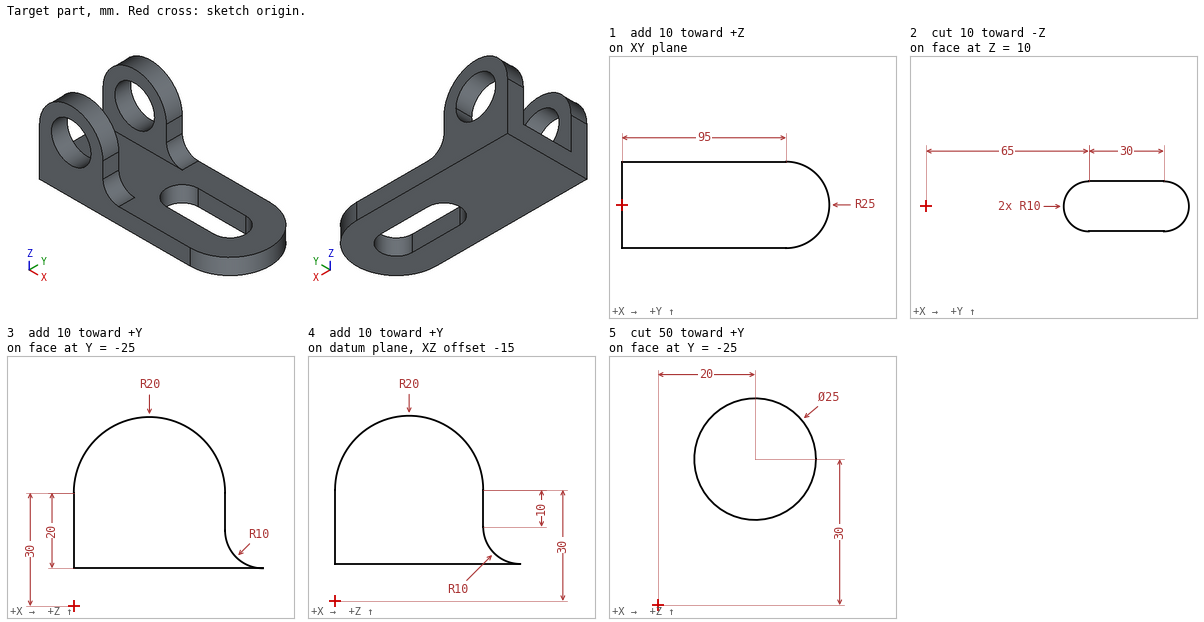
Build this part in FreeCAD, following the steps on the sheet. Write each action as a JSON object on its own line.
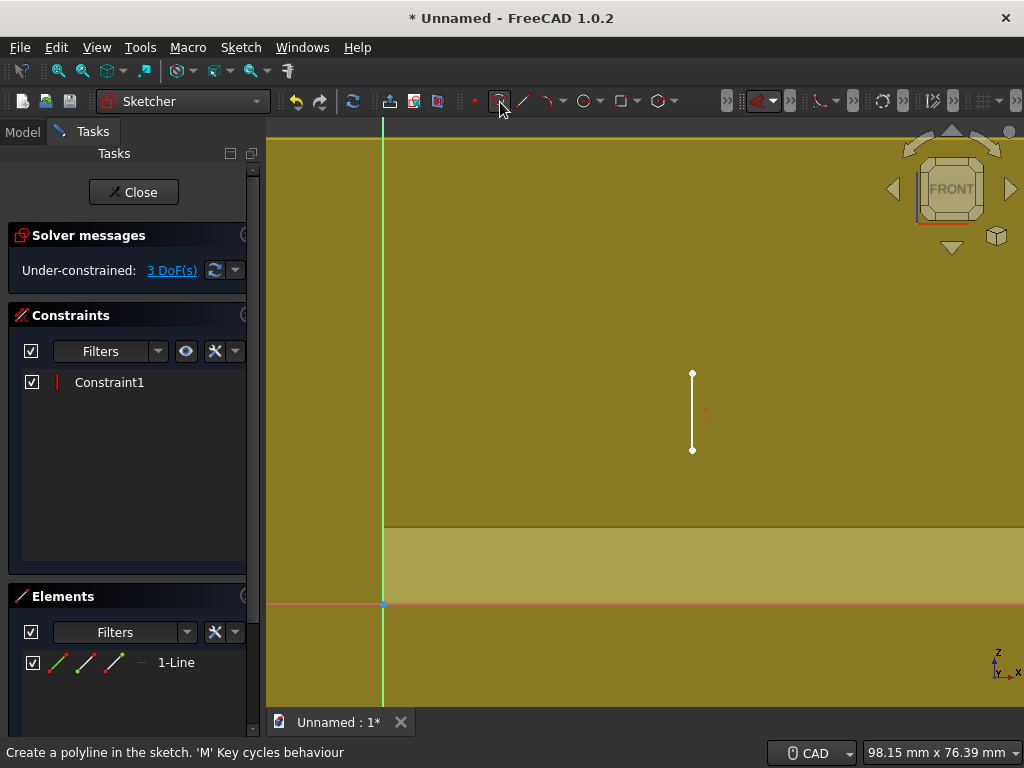
{"action": "left_click", "coordinate": [769, 527]}
{"action": "left_click", "coordinate": [383, 527]}
{"action": "left_click", "coordinate": [392, 373]}
{"action": "right_click", "coordinate": [392, 373]}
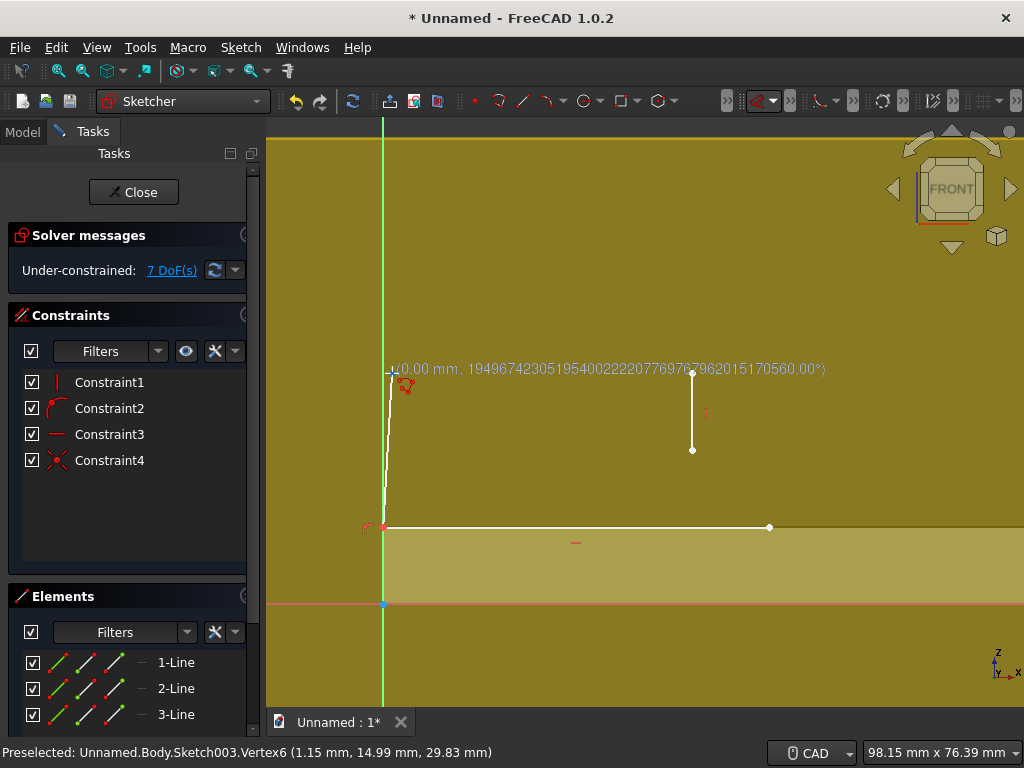
{"action": "left_click", "coordinate": [548, 102]}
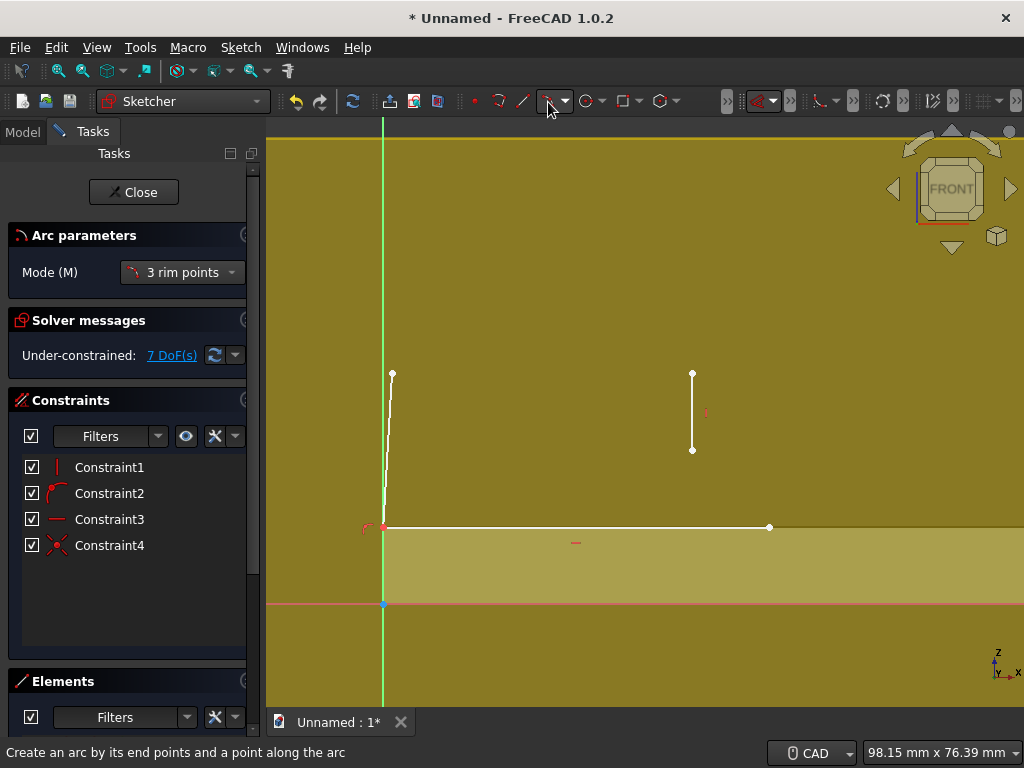
{"action": "left_click", "coordinate": [692, 451]}
{"action": "left_click", "coordinate": [769, 528]}
{"action": "left_click", "coordinate": [715, 505]}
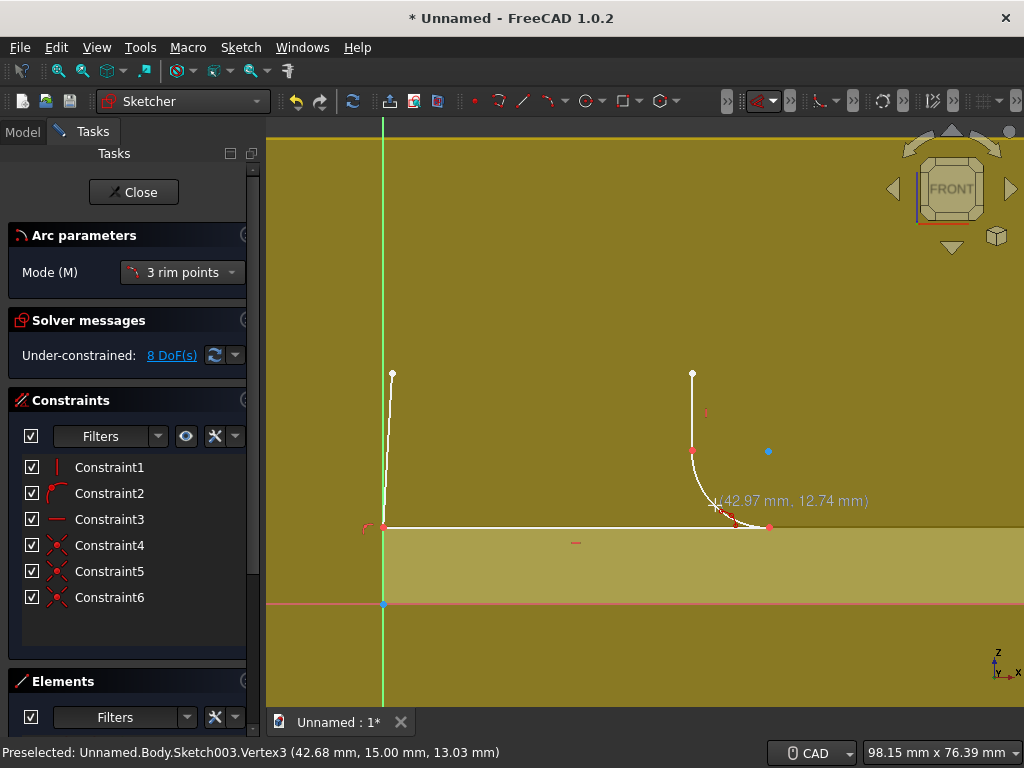
{"action": "left_click", "coordinate": [392, 374]}
{"action": "left_click", "coordinate": [692, 374]}
{"action": "left_click", "coordinate": [538, 218]}
{"action": "key", "text": "Escape"}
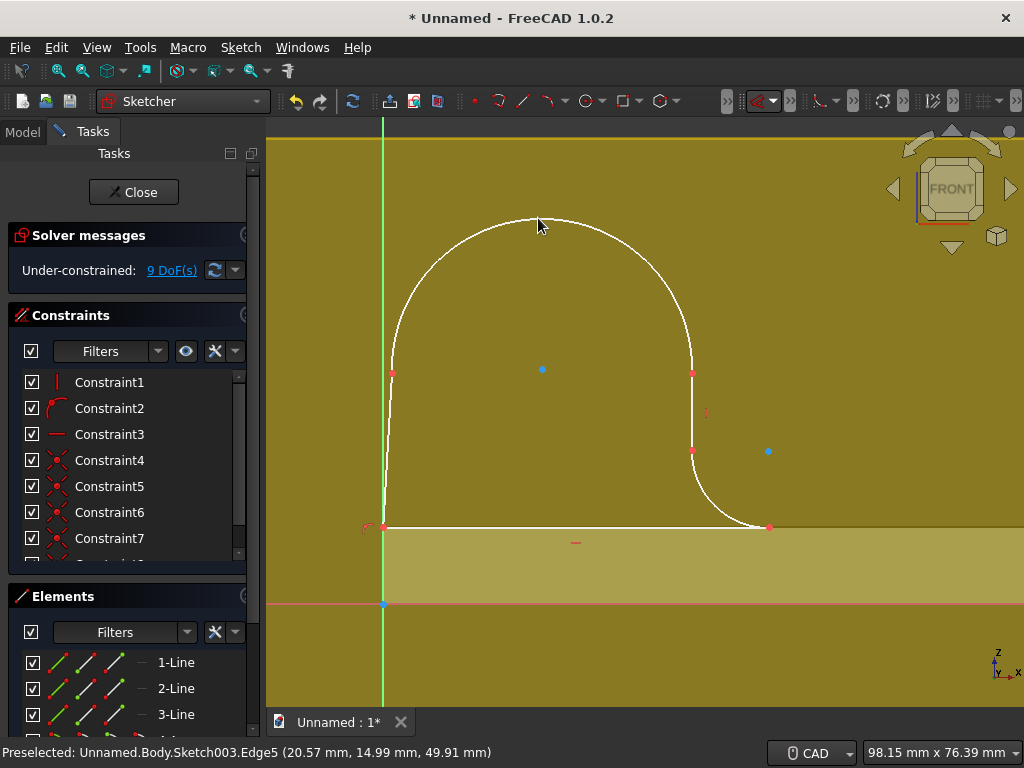
{"action": "left_click", "coordinate": [692, 397]}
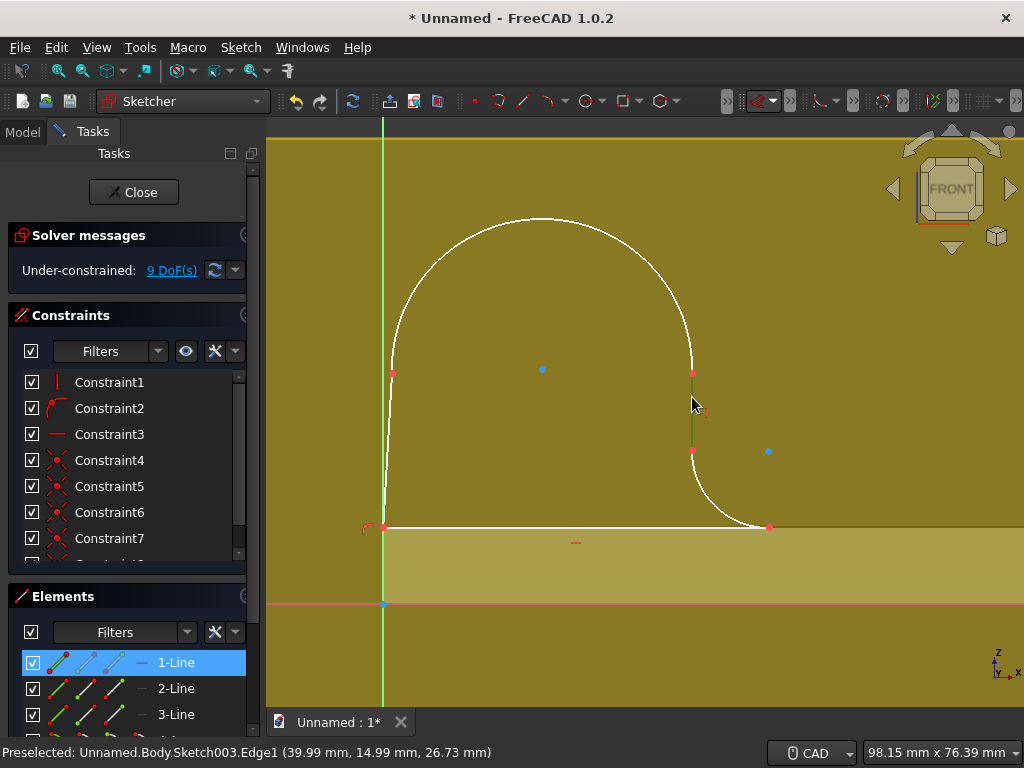
{"action": "left_click", "coordinate": [700, 486]}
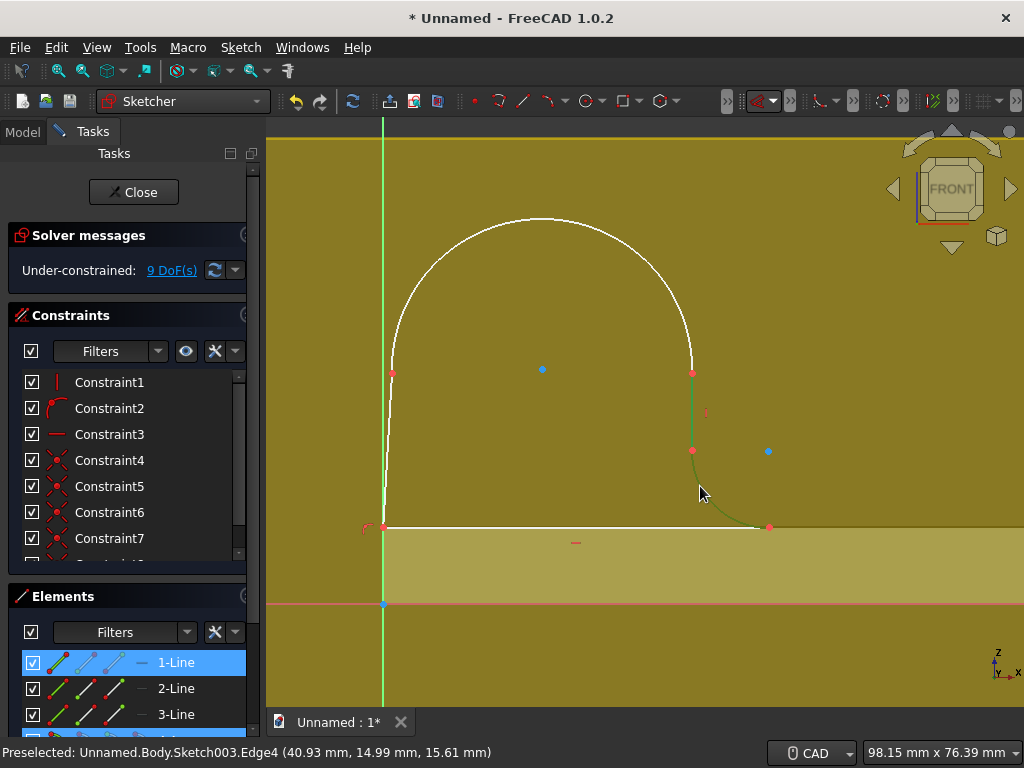
{"action": "key", "text": "t"}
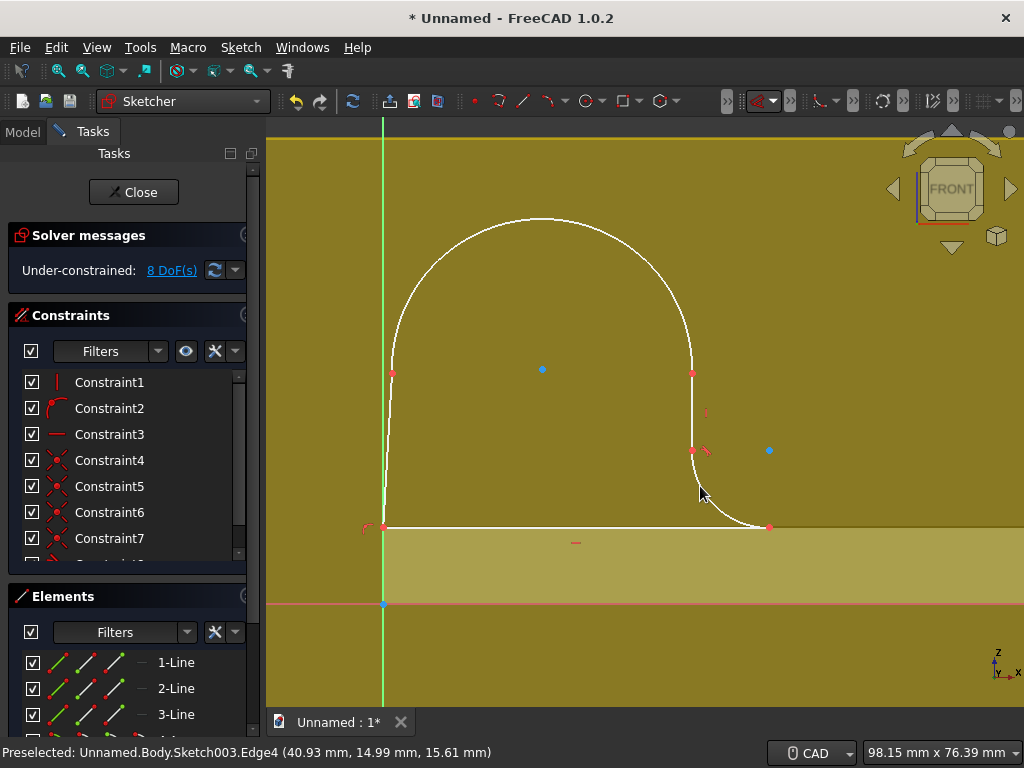
{"action": "left_click", "coordinate": [692, 397]}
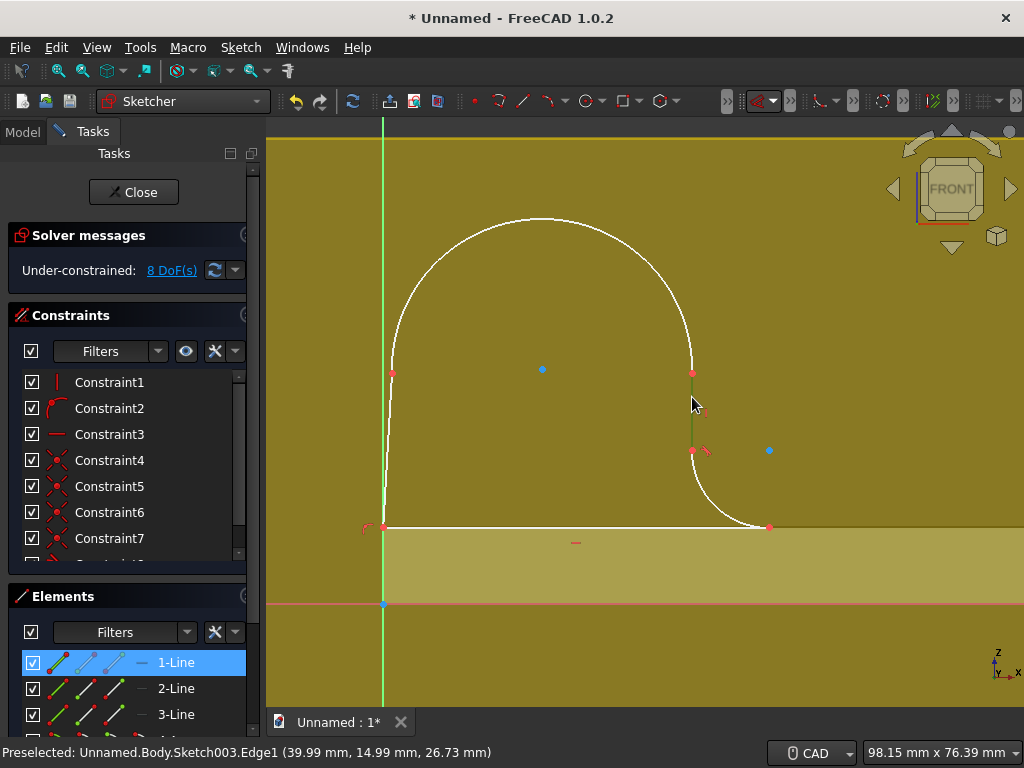
{"action": "left_click", "coordinate": [632, 249]}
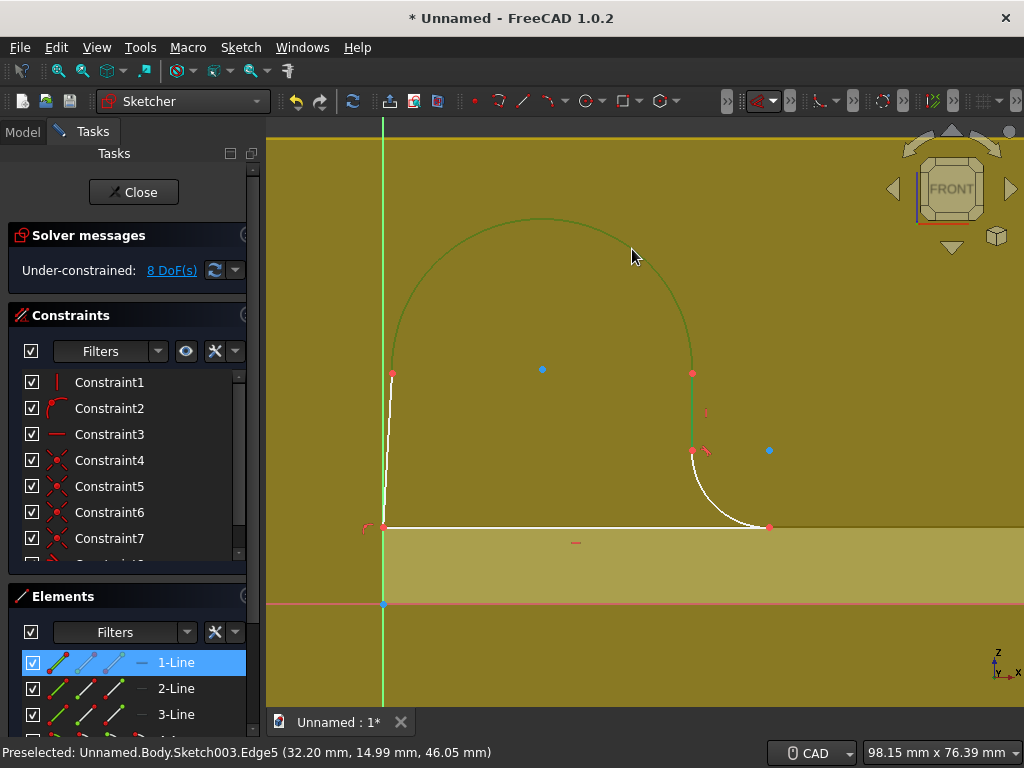
{"action": "key", "text": "t"}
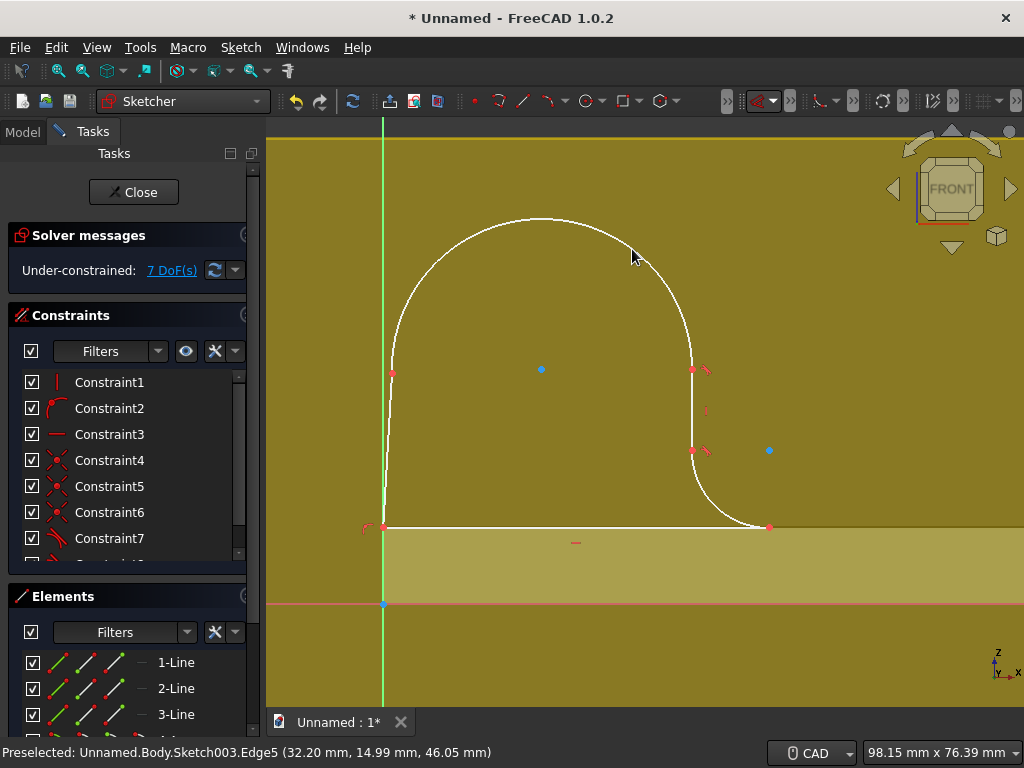
{"action": "left_click", "coordinate": [653, 528]}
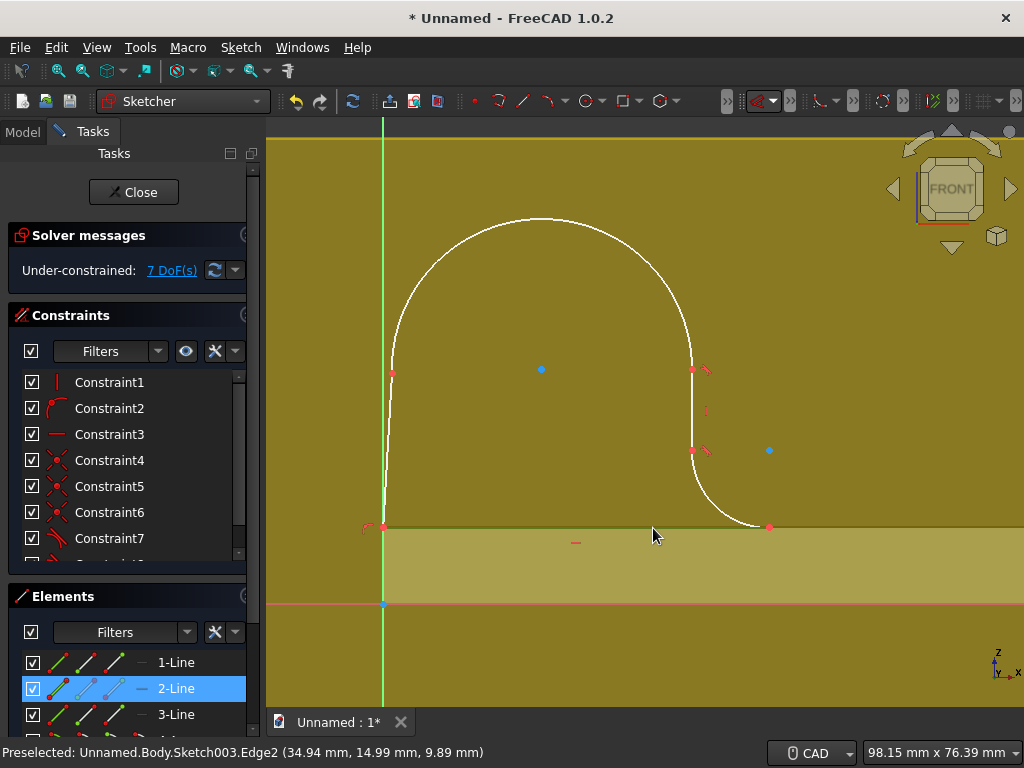
{"action": "left_click", "coordinate": [700, 486]}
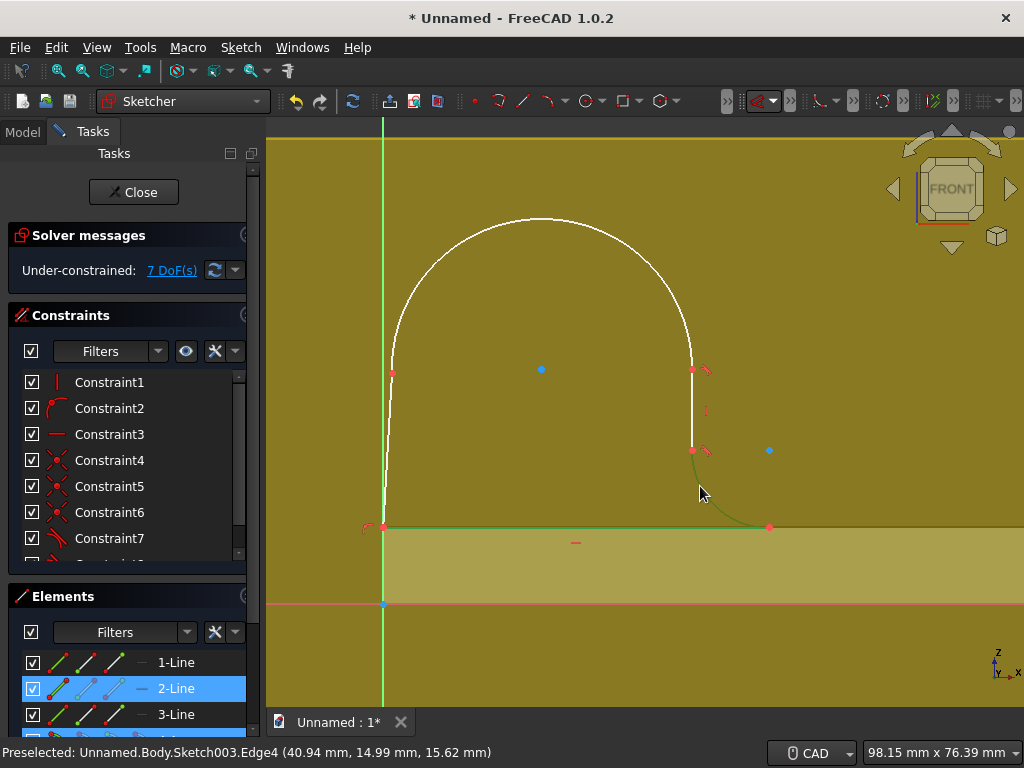
{"action": "key", "text": "t"}